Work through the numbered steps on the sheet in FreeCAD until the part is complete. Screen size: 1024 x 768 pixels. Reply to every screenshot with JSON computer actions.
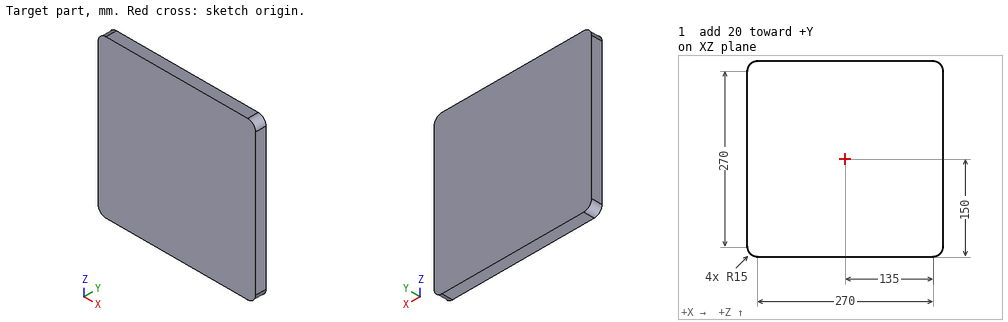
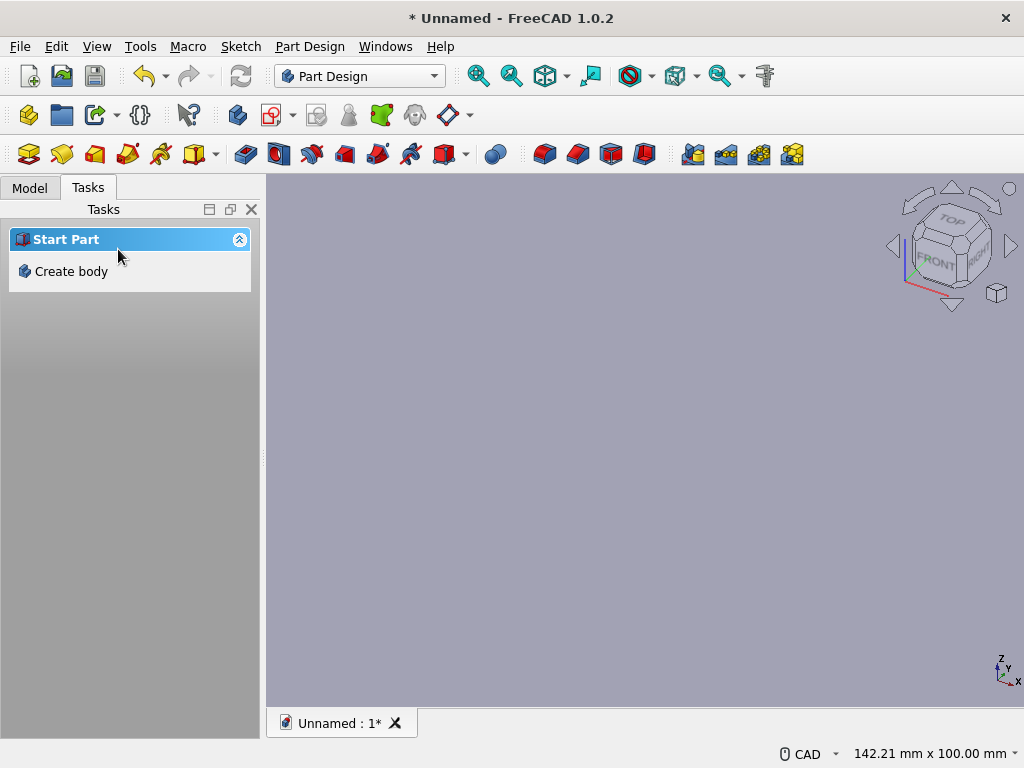
{"action": "key", "text": "0"}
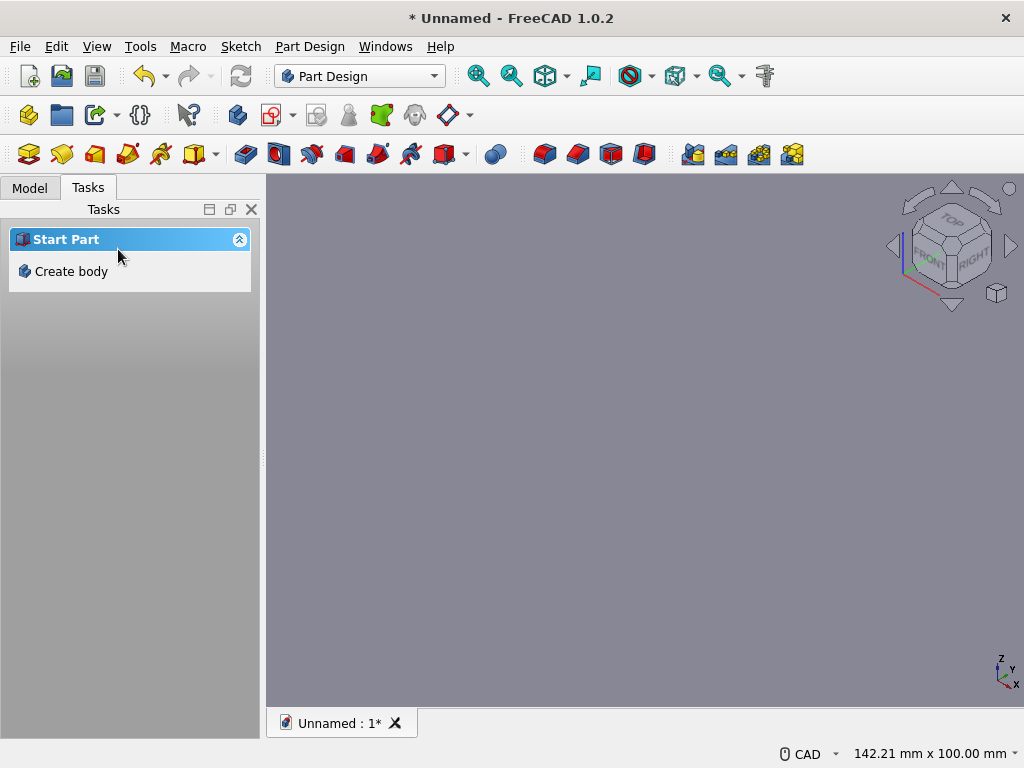
{"action": "left_click", "coordinate": [479, 76]}